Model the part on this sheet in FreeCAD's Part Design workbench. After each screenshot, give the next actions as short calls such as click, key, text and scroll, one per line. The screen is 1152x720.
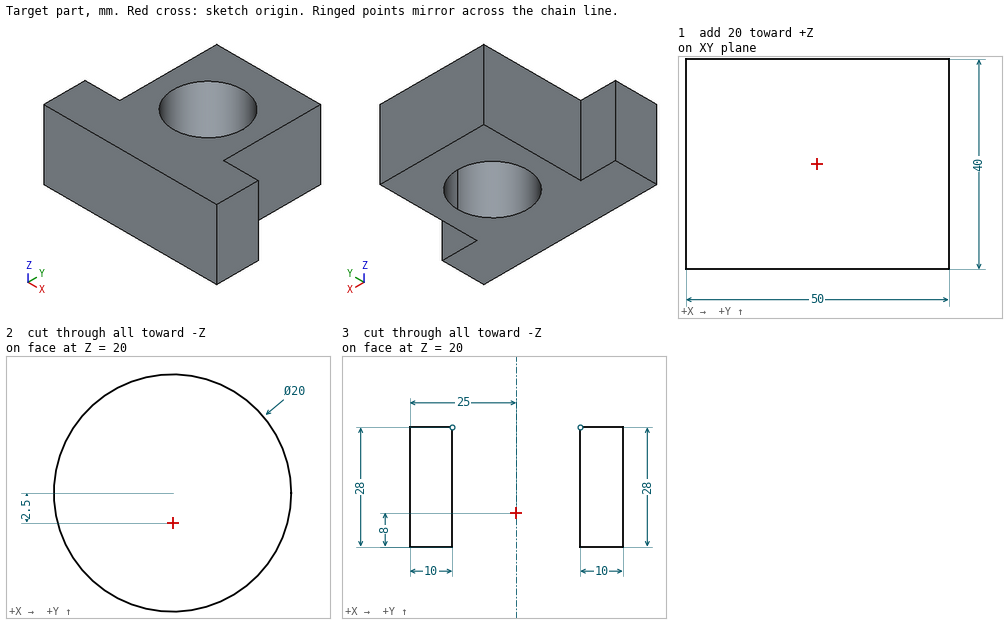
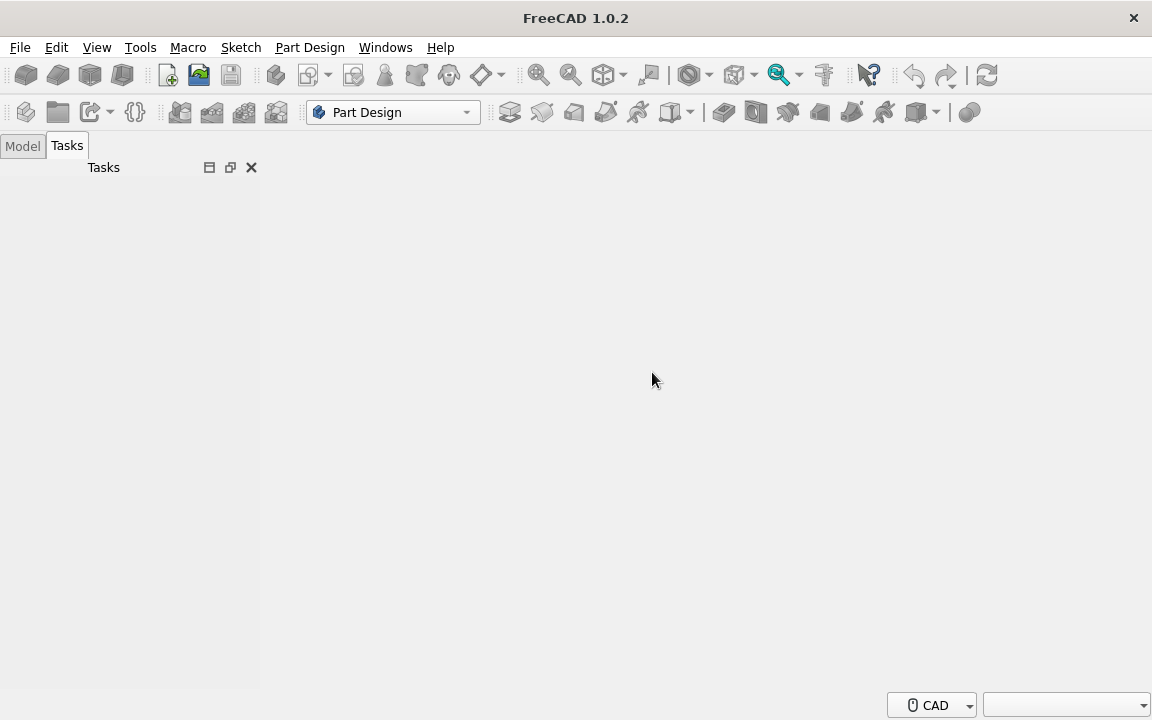
key(ctrl+n)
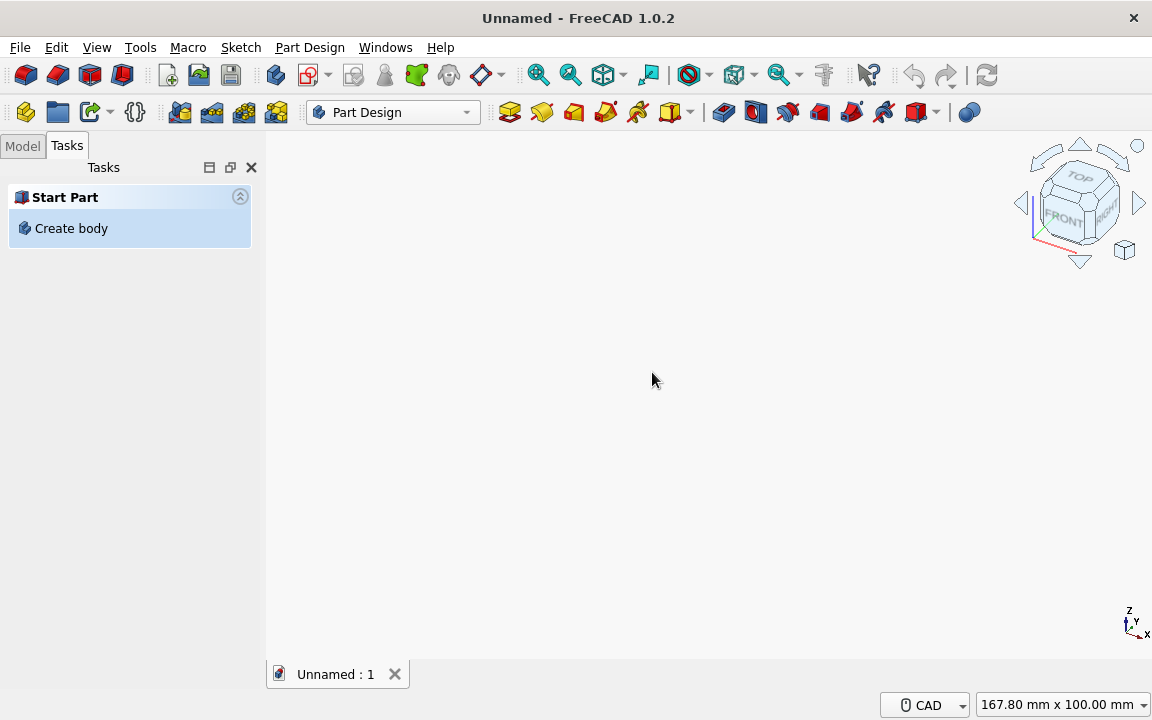
click(308, 76)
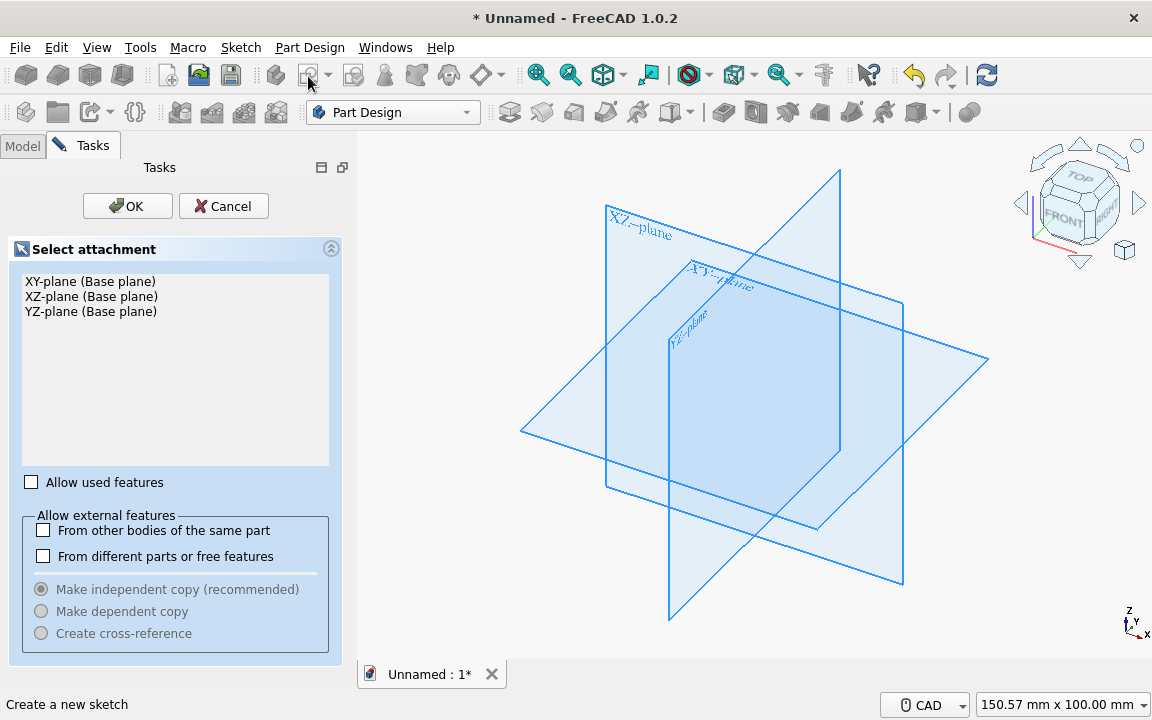
click(82, 282)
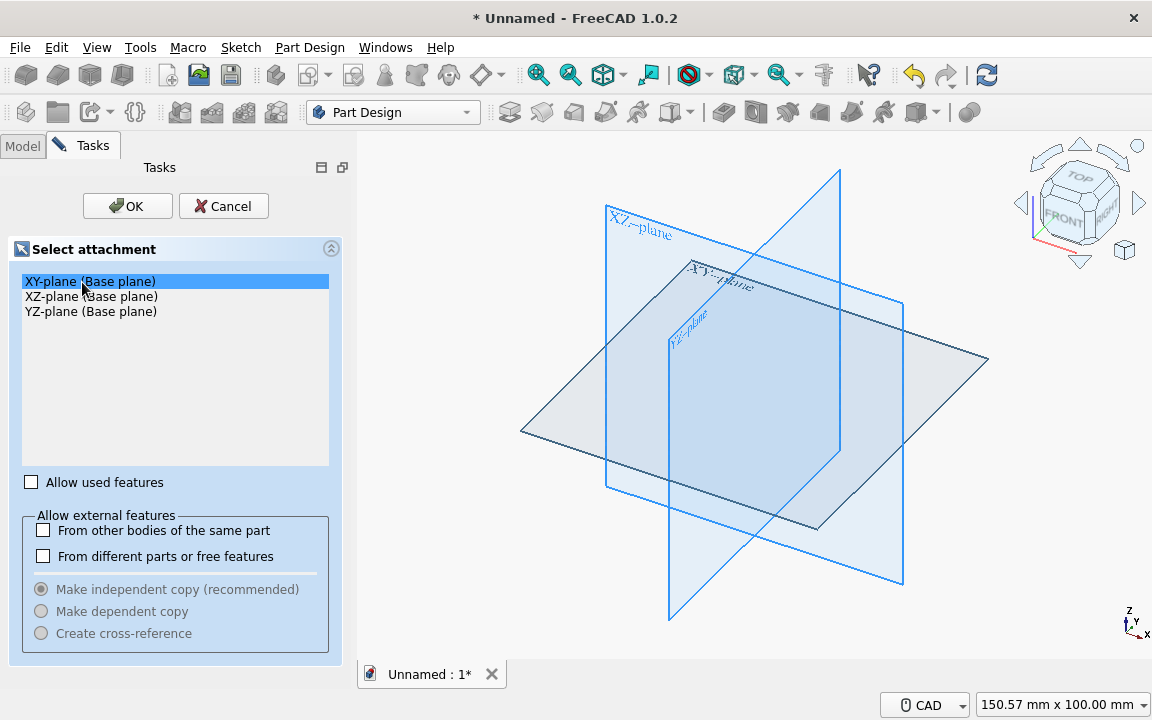
click(128, 206)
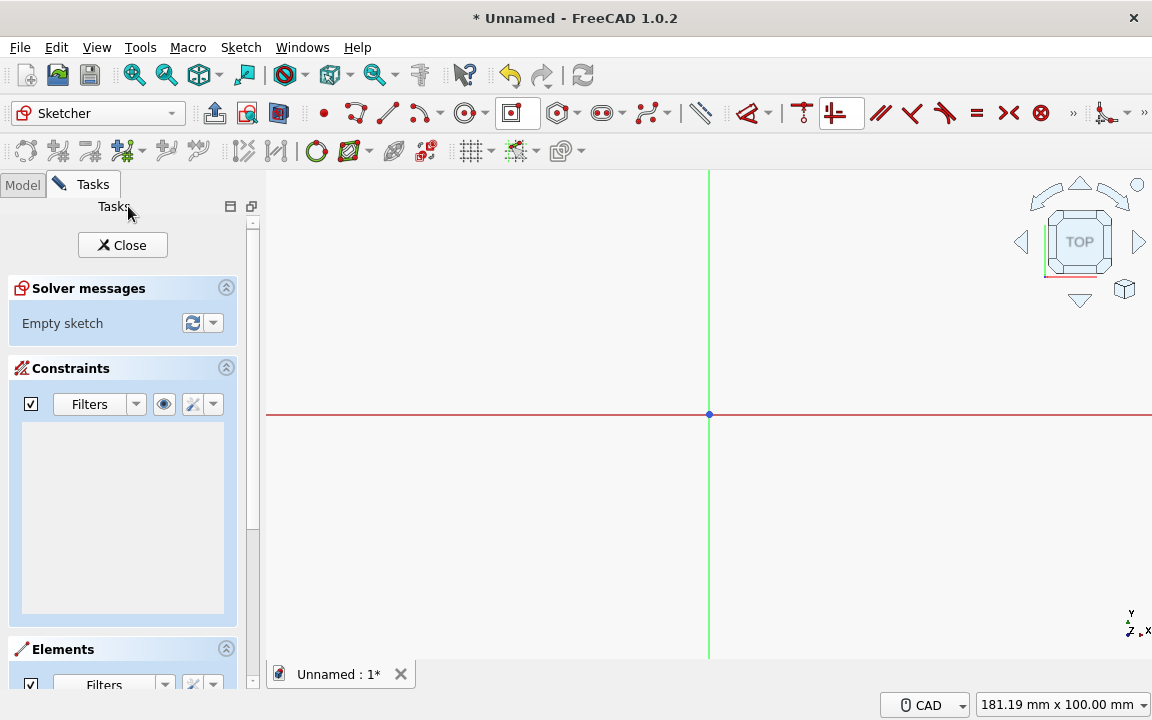
scroll(848, 414, up, 2)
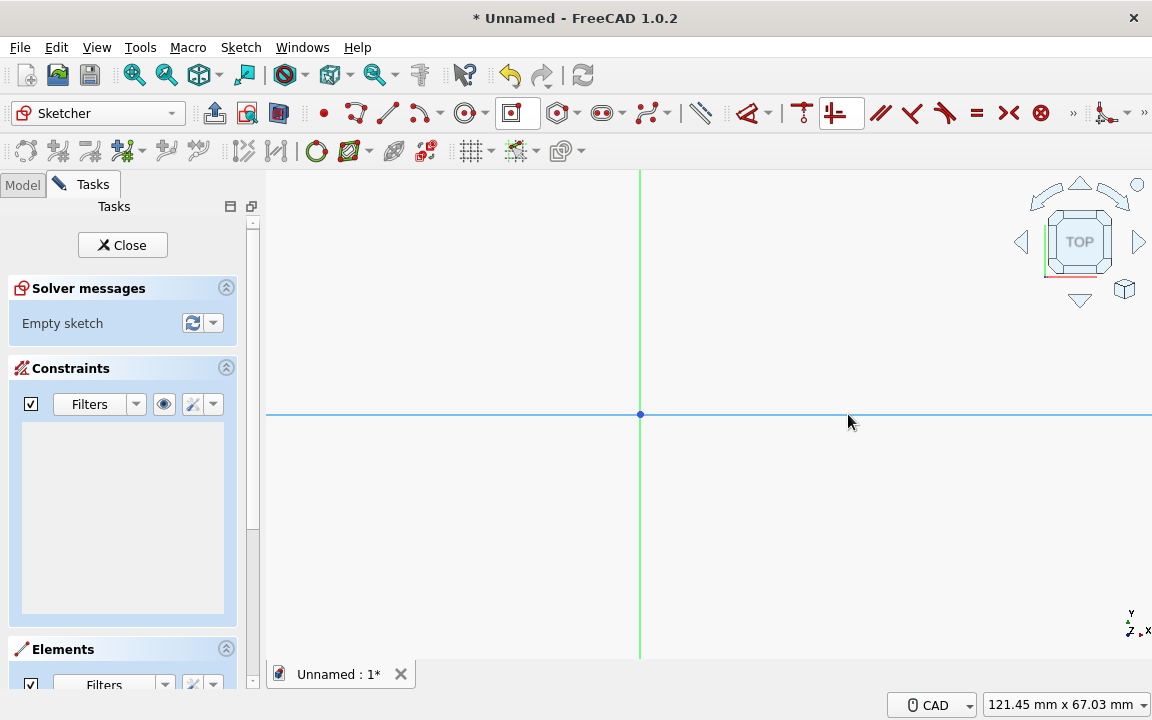
click(512, 114)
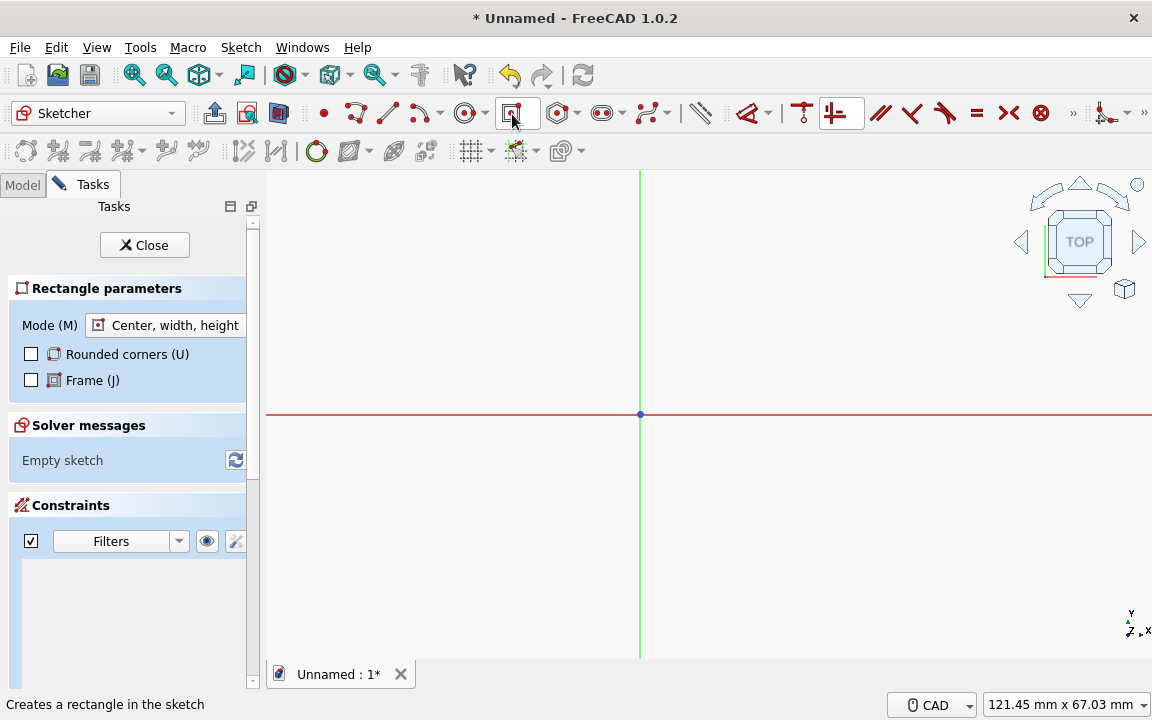
click(640, 414)
move(823, 269)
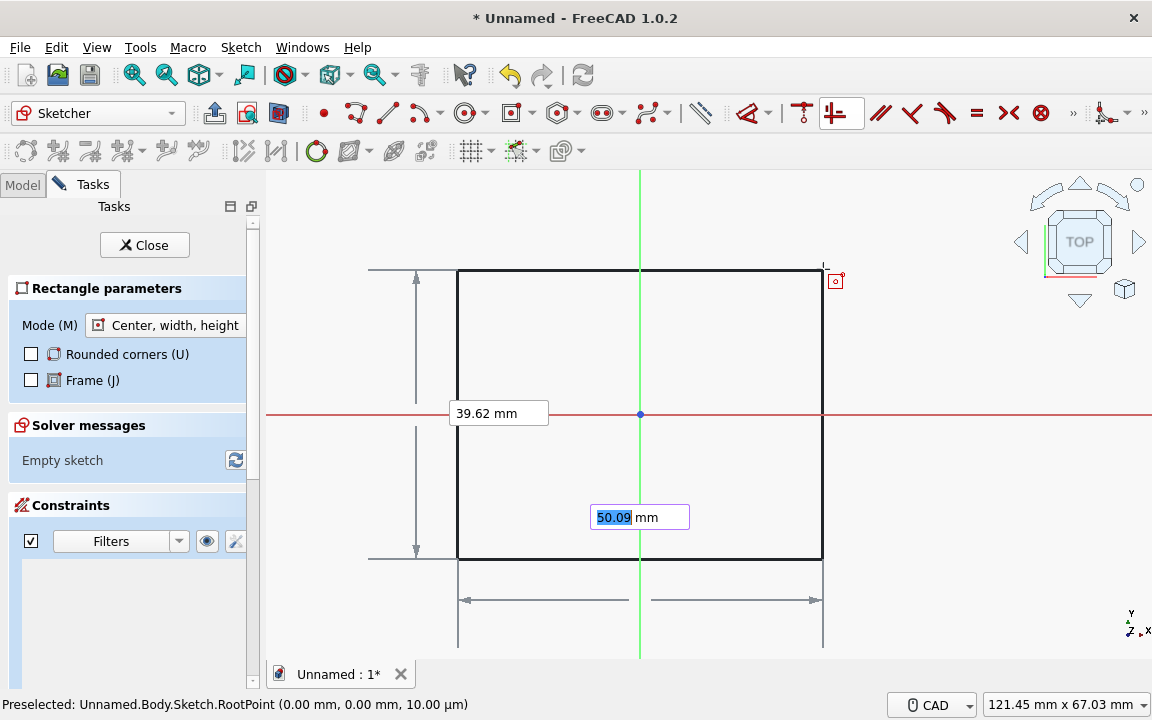
text(50)
key(Tab)
text(40)
key(Return)
key(Escape)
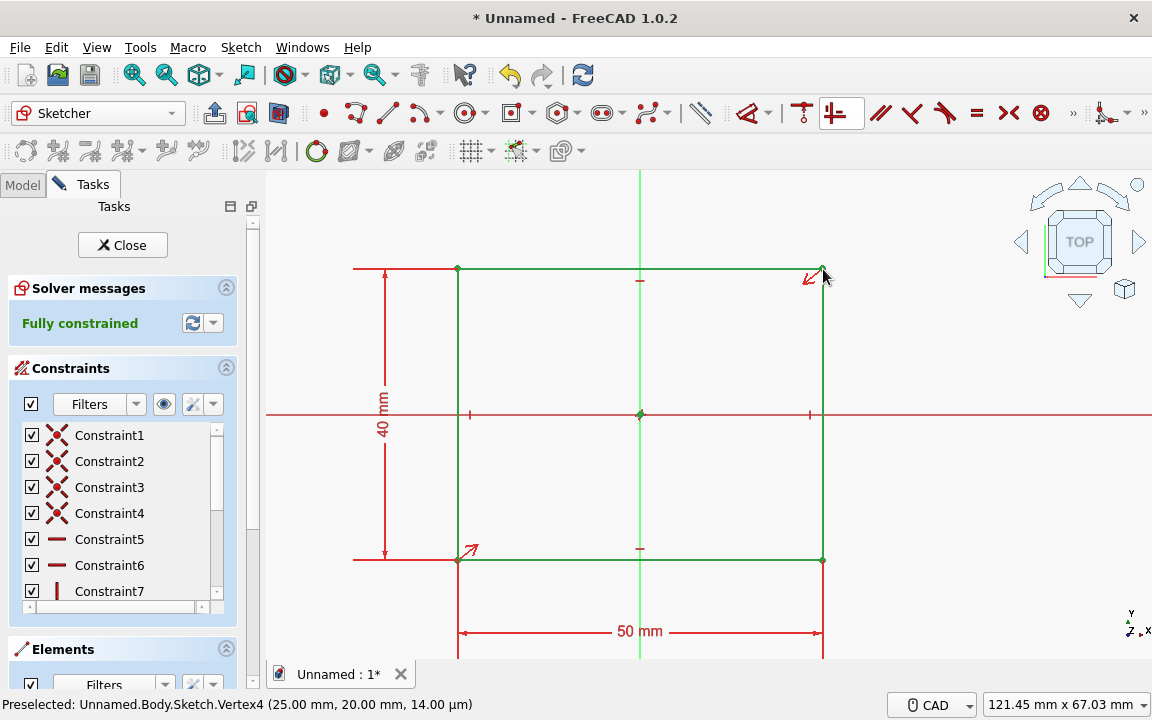
click(123, 245)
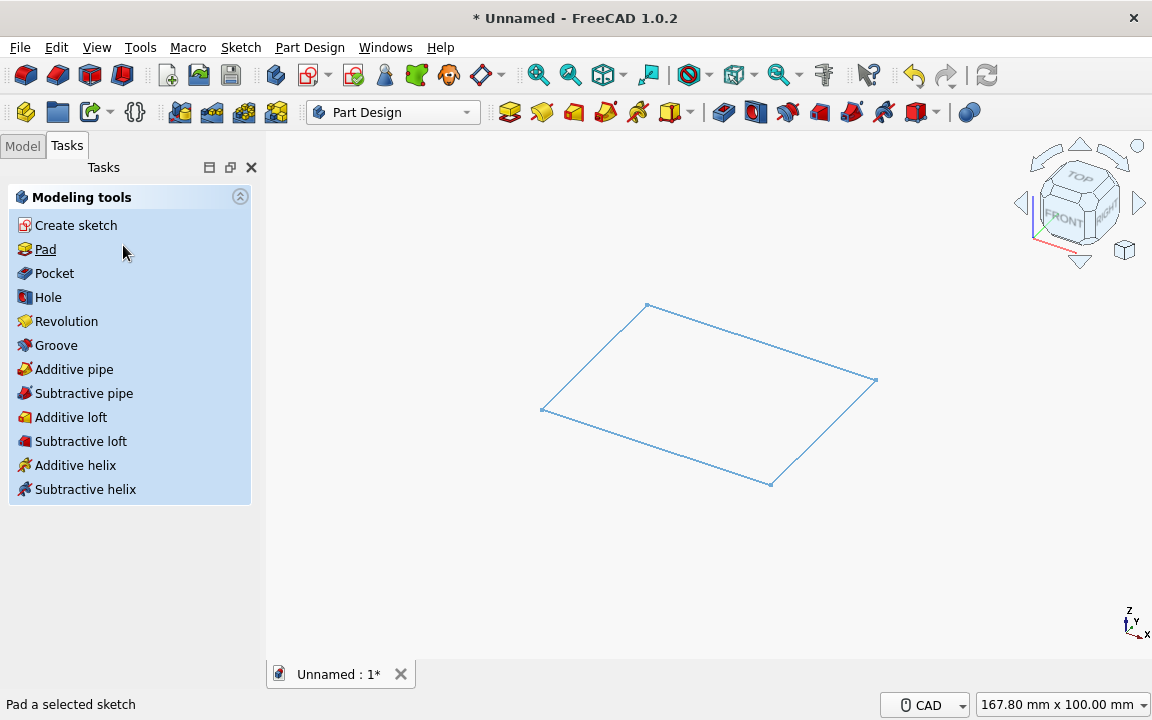
click(510, 112)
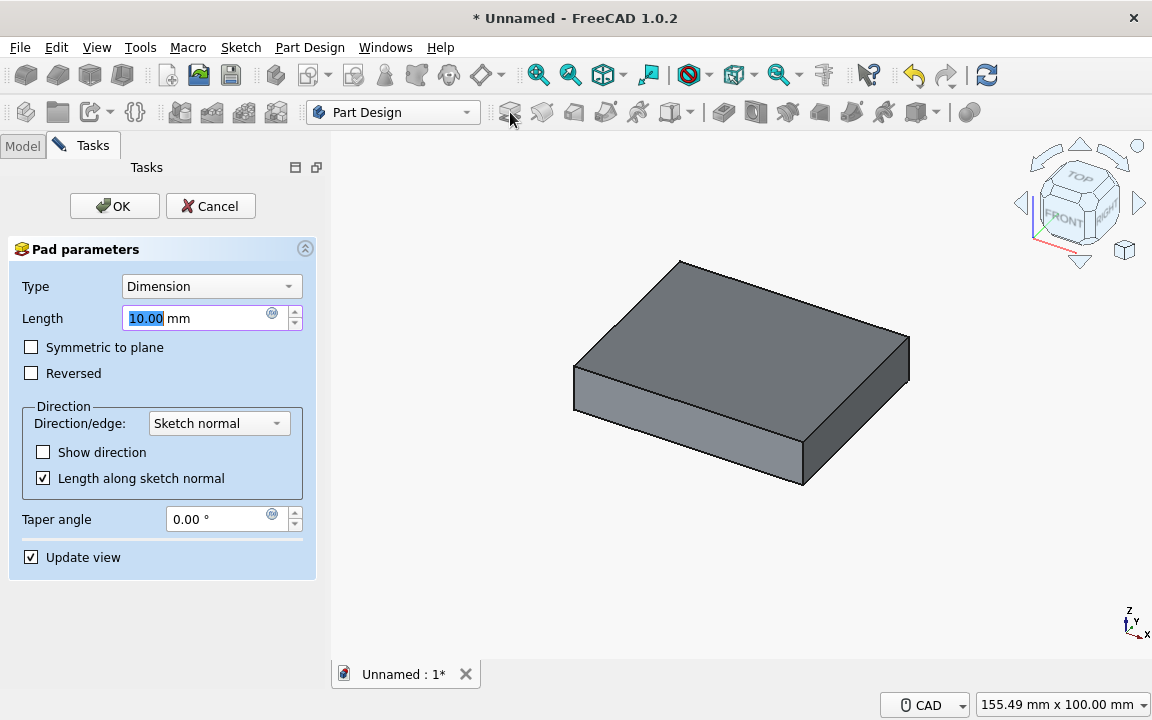
text(20)
key(Tab)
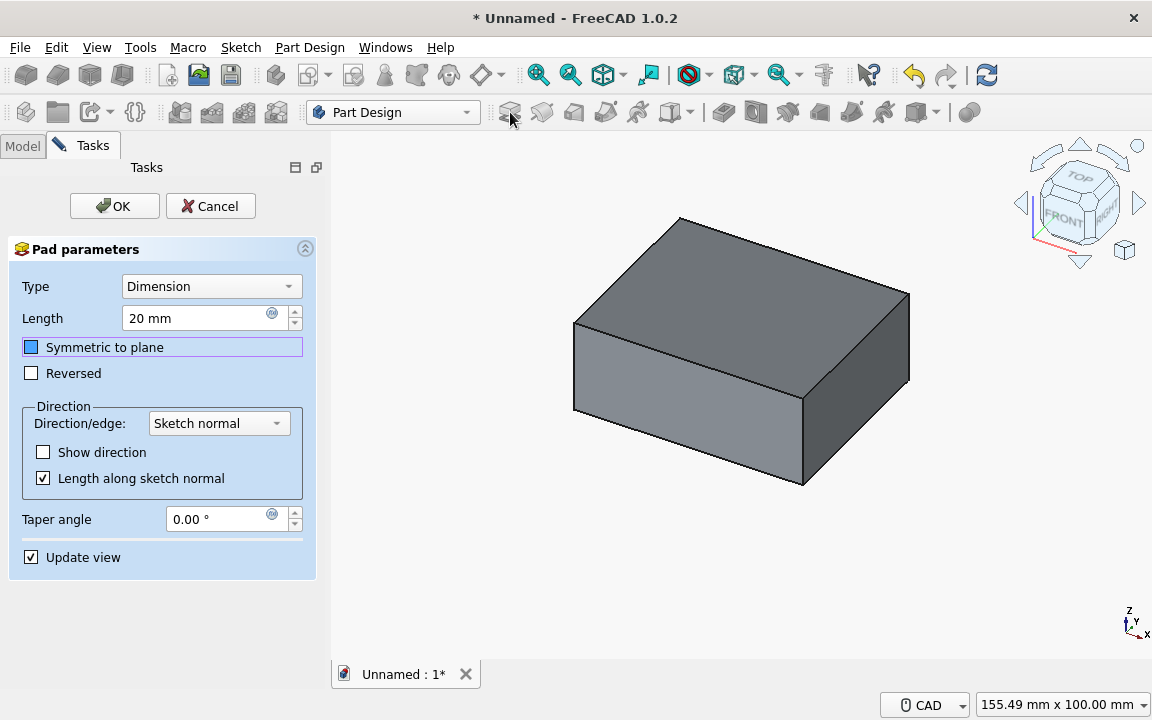
click(115, 206)